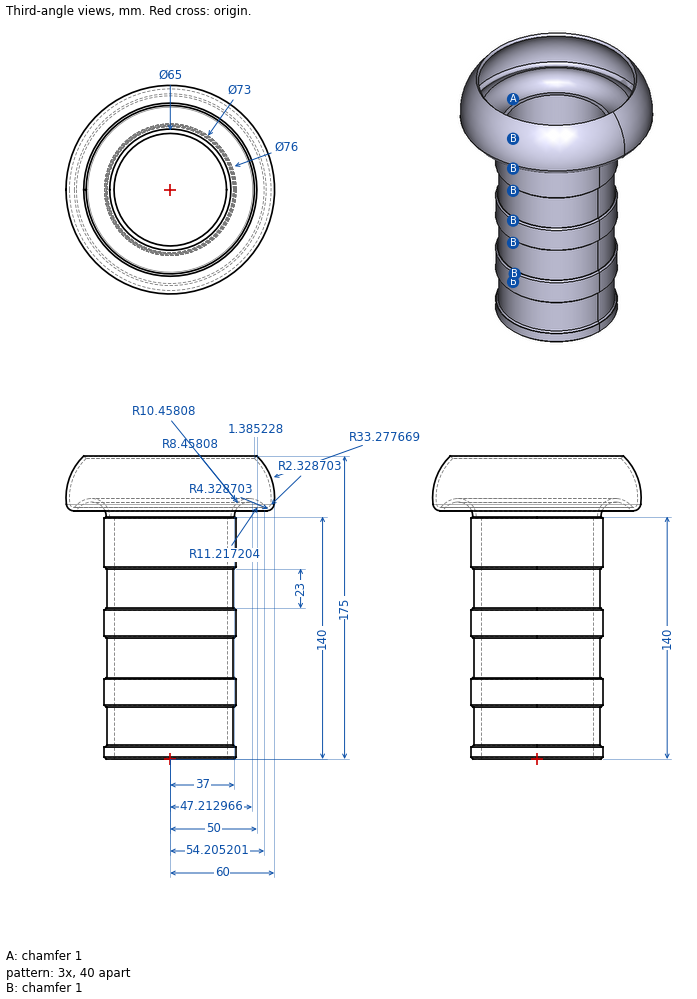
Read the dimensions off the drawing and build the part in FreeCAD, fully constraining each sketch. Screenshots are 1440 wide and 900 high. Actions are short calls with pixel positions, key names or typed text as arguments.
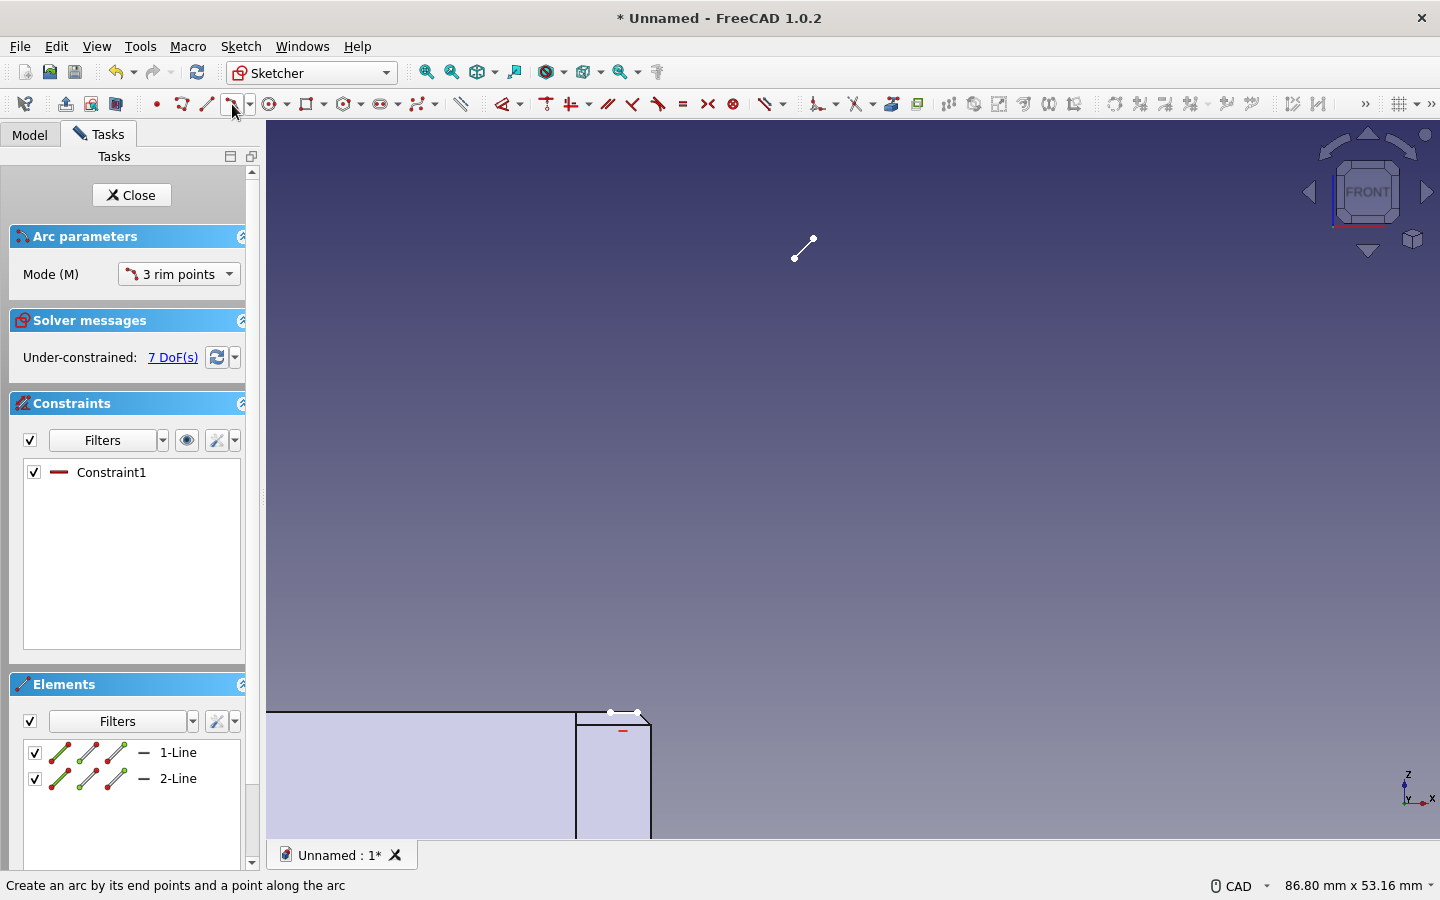
click(813, 239)
click(948, 616)
click(925, 411)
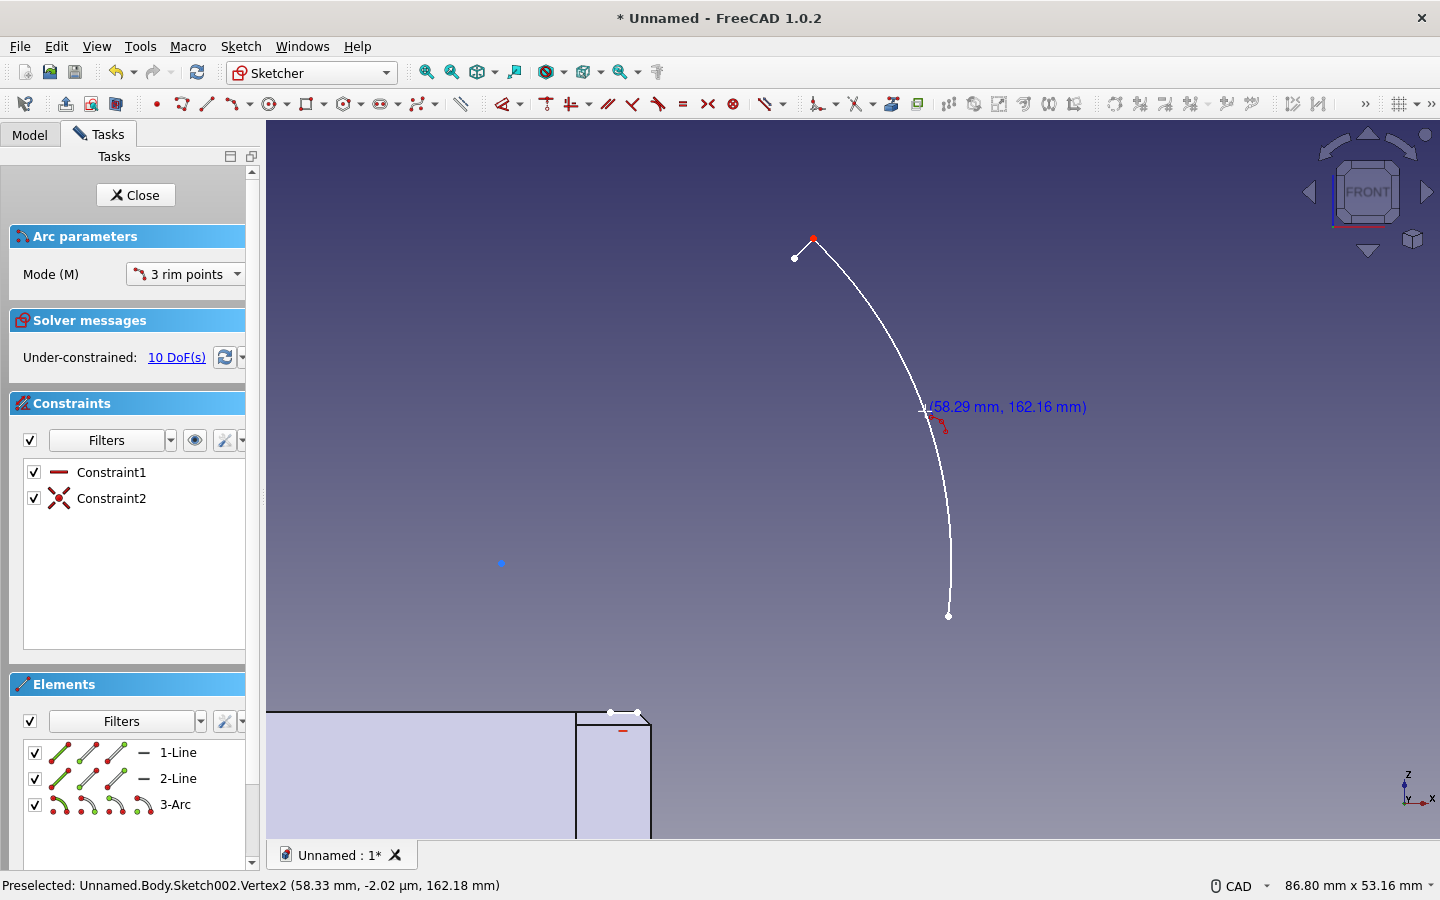
click(948, 617)
click(870, 664)
click(921, 659)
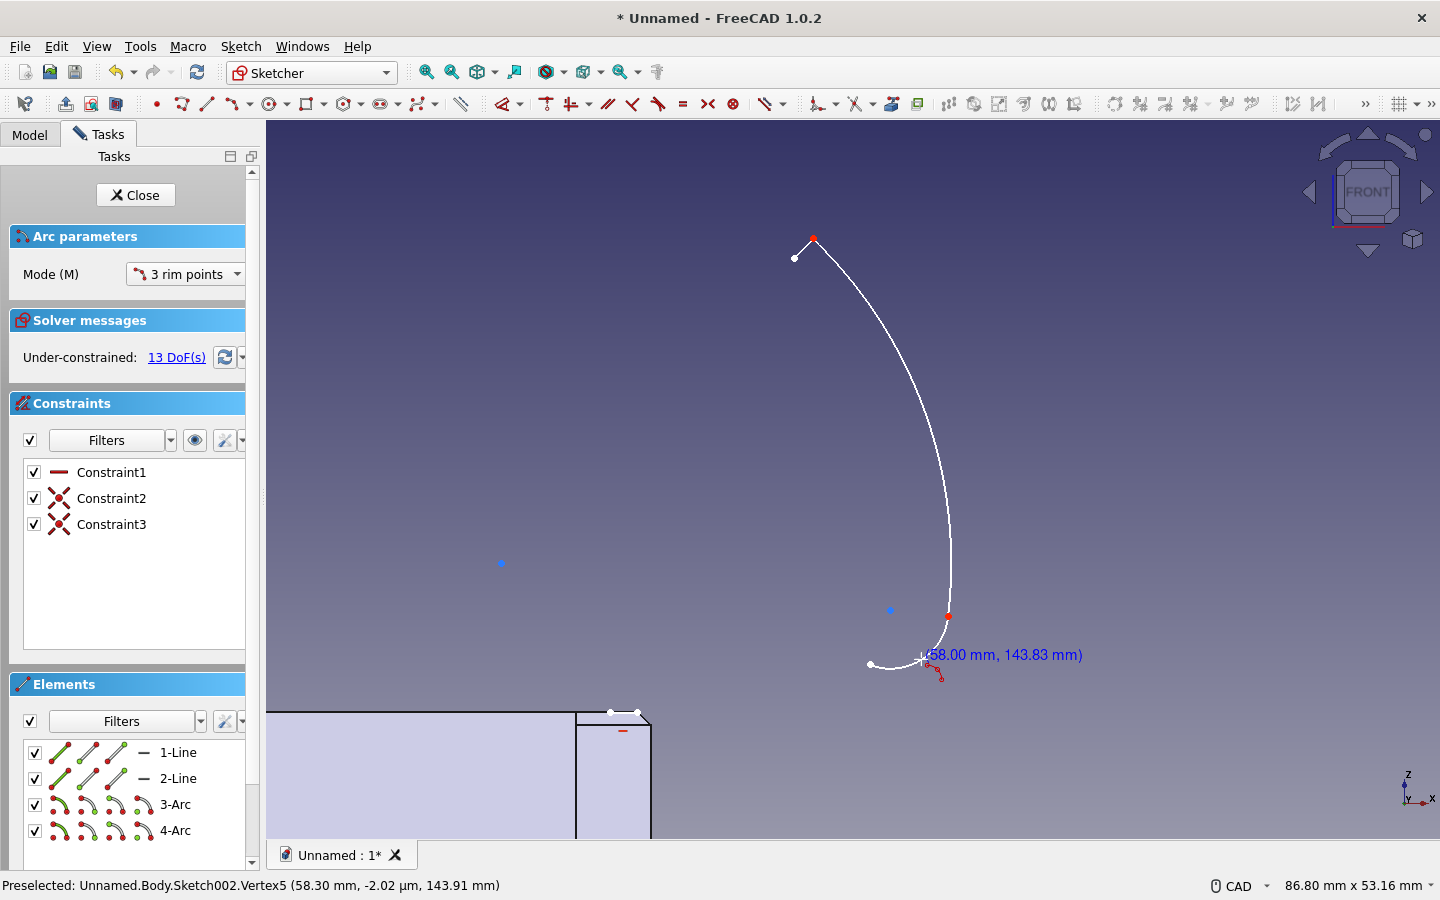
click(870, 665)
click(775, 600)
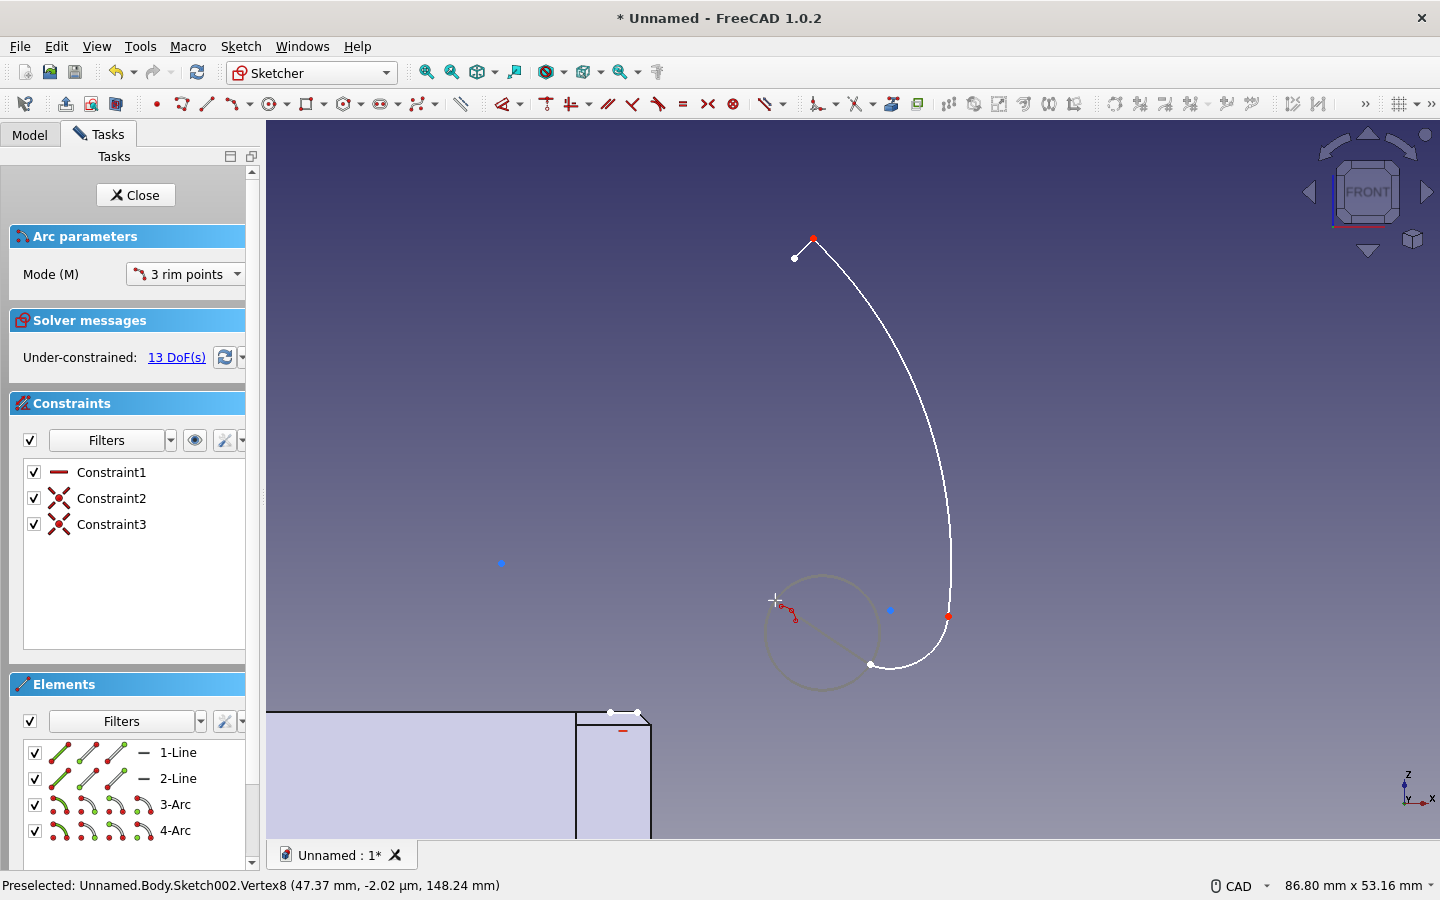
scroll(829, 623, up, 2)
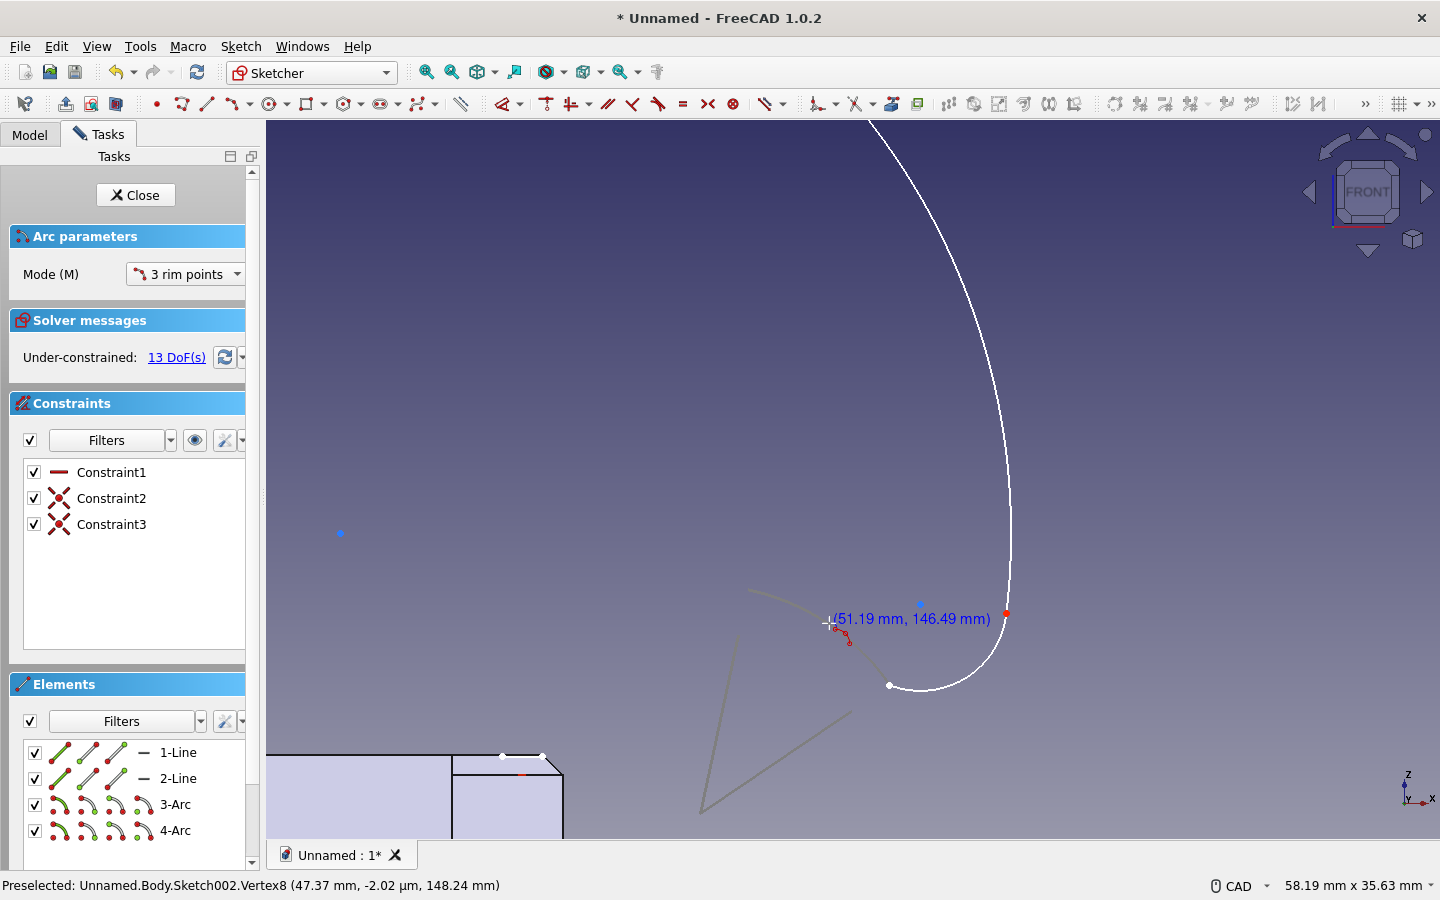
click(828, 622)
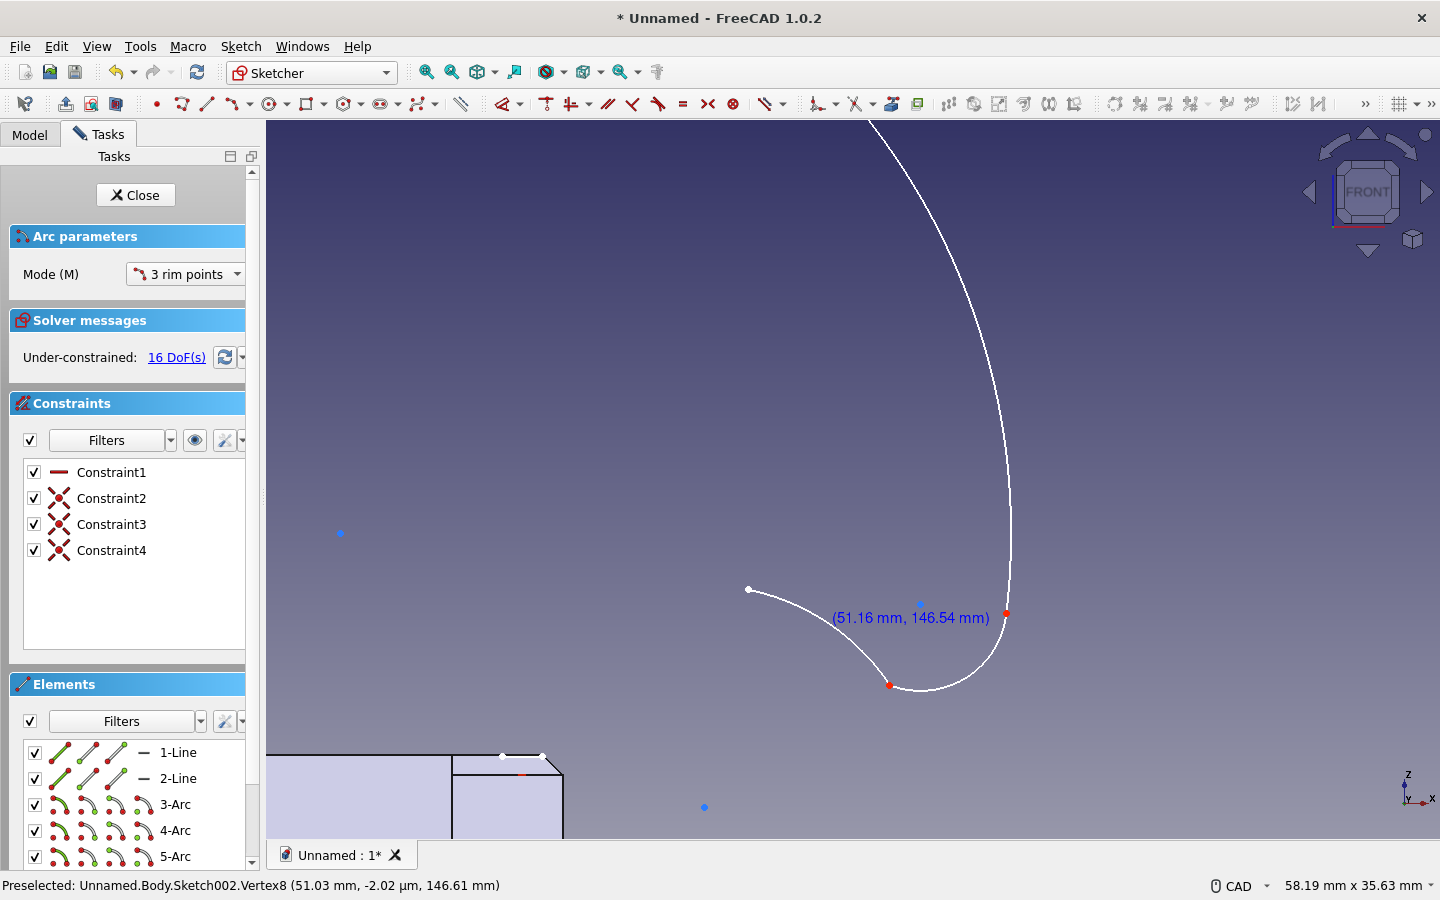
click(748, 590)
click(542, 757)
click(606, 622)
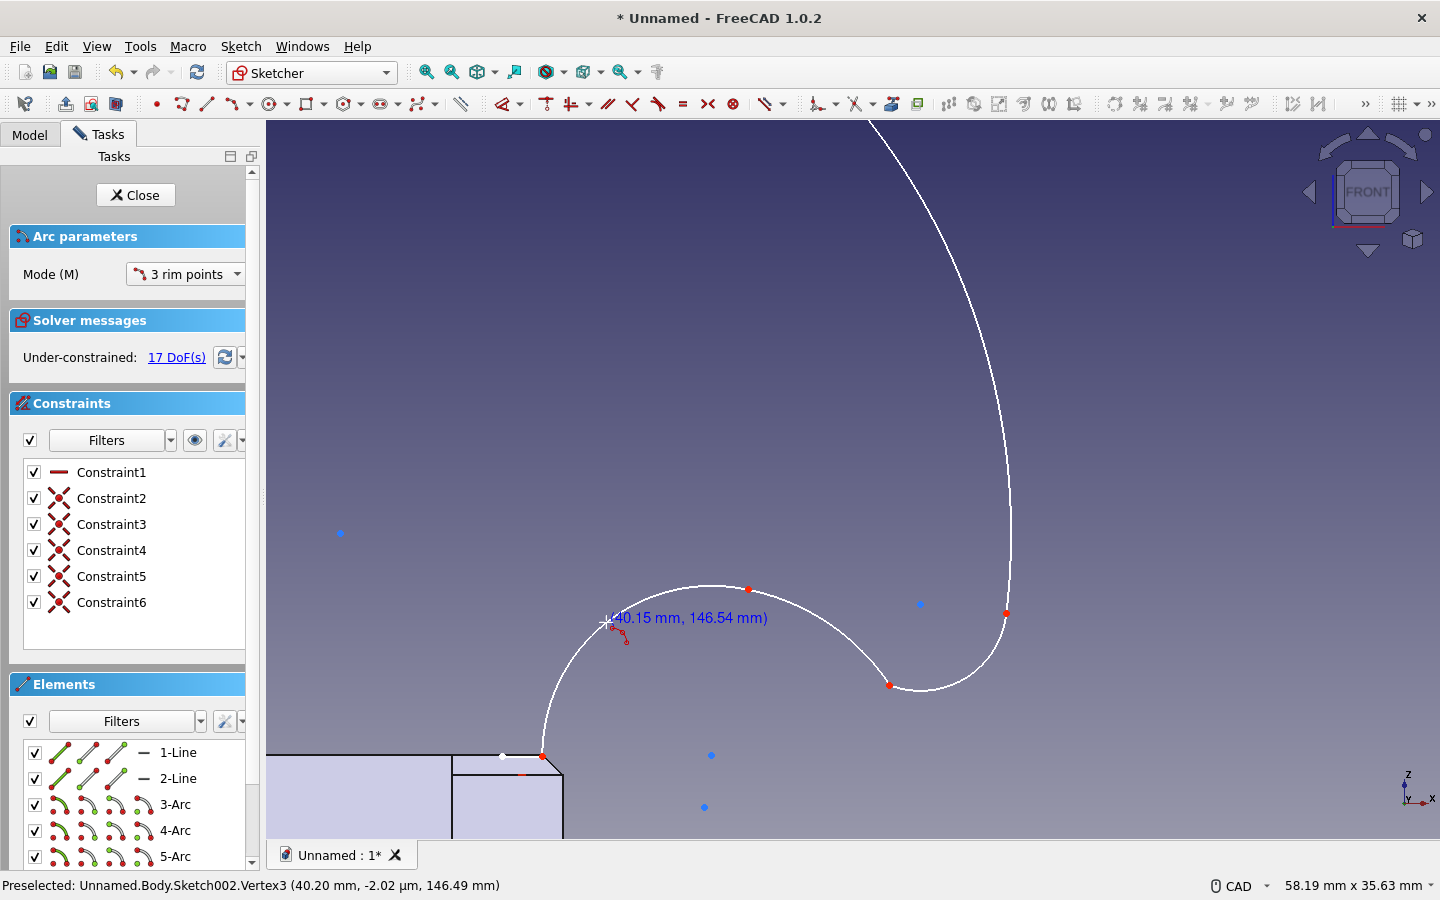
click(502, 757)
click(757, 549)
click(580, 591)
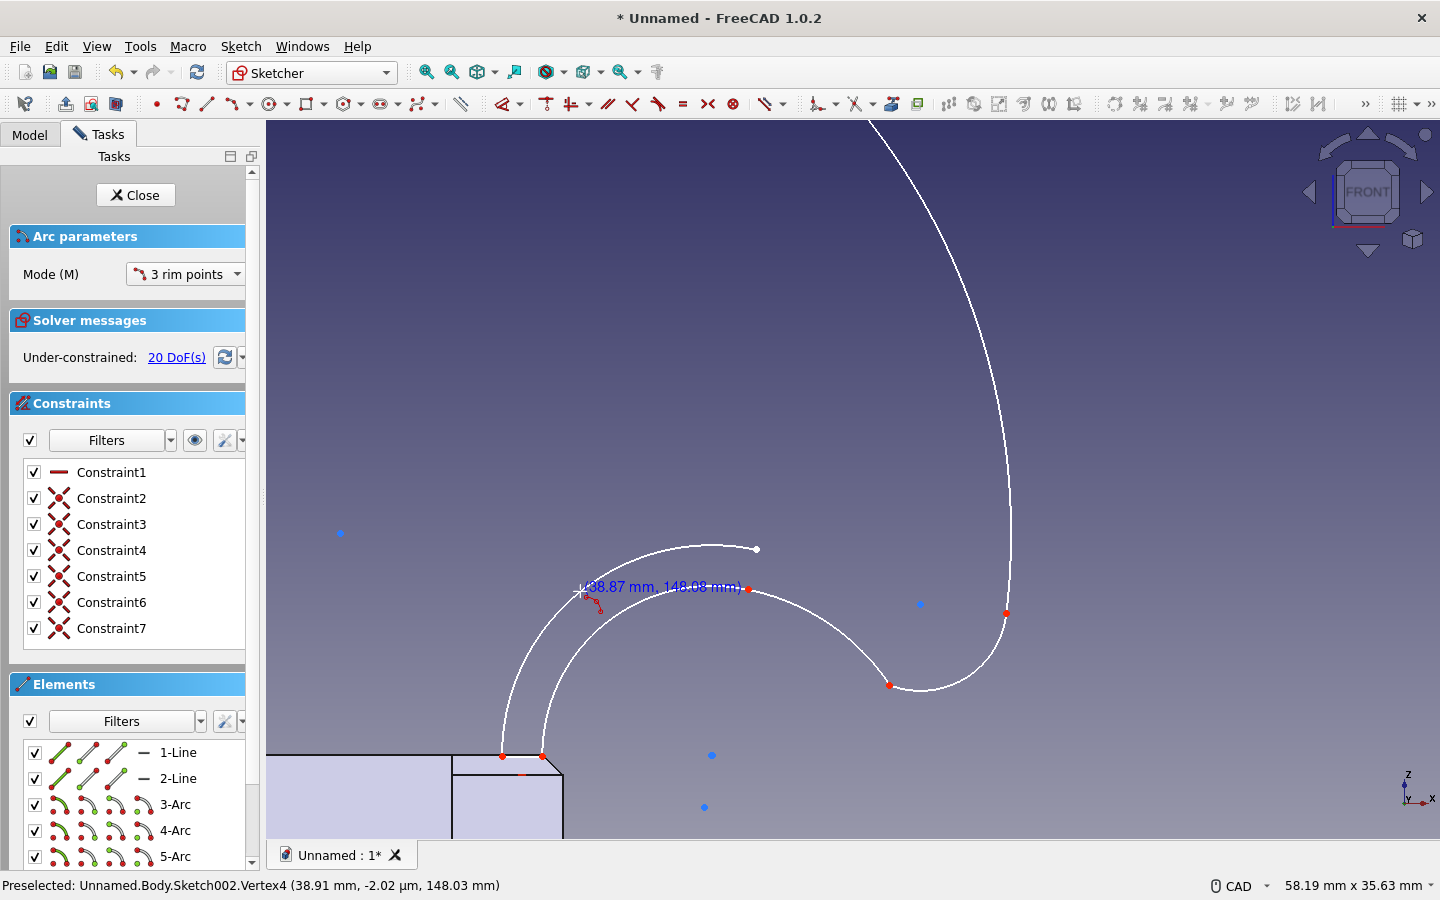
click(757, 550)
click(914, 648)
click(844, 584)